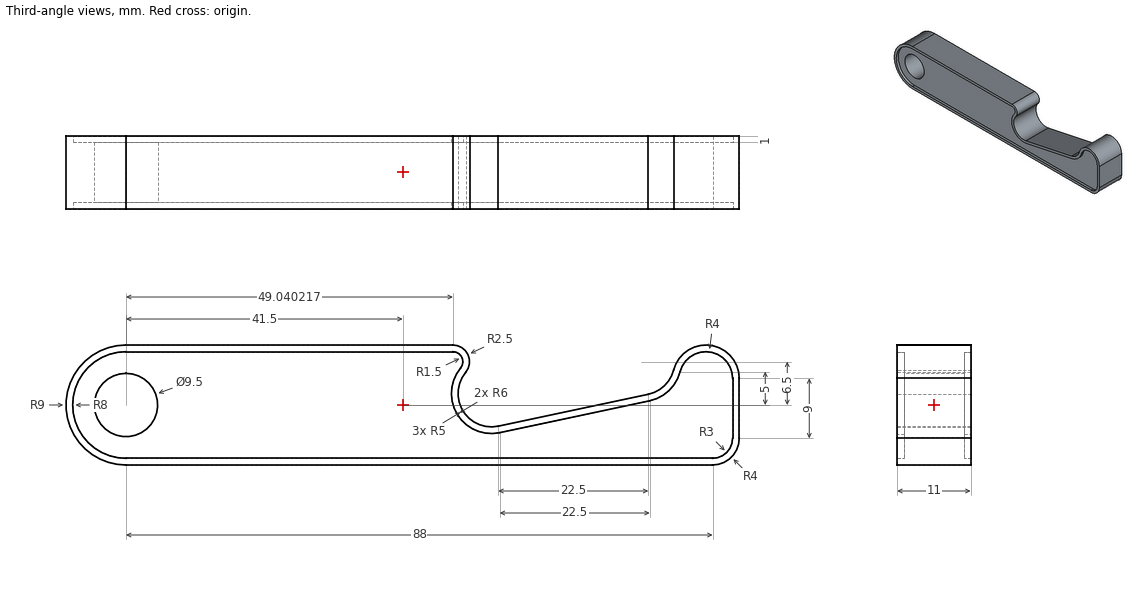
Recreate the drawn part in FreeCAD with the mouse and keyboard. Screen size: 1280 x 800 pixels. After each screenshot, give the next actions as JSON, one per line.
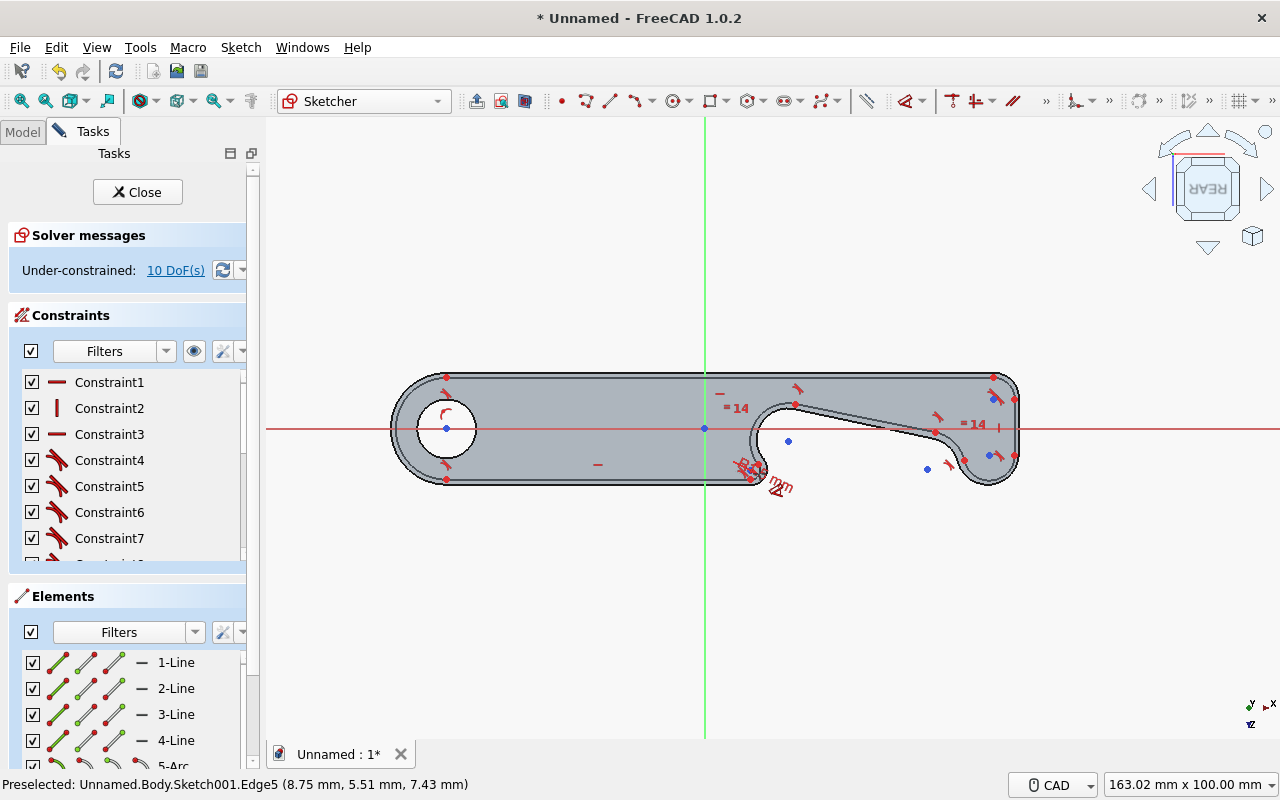
{"action": "left_click", "coordinate": [769, 409]}
{"action": "left_click", "coordinate": [728, 406]}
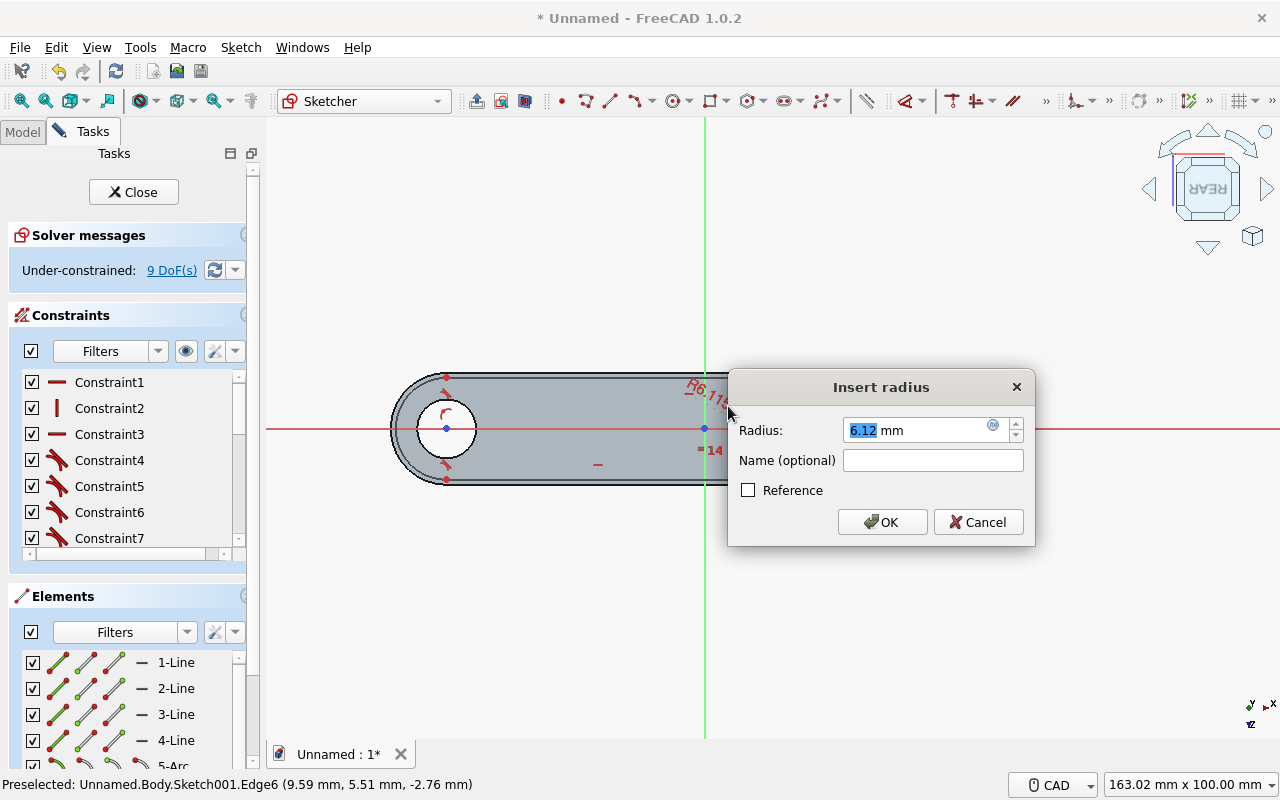
{"action": "type", "text": "6"}
{"action": "key", "text": "Return"}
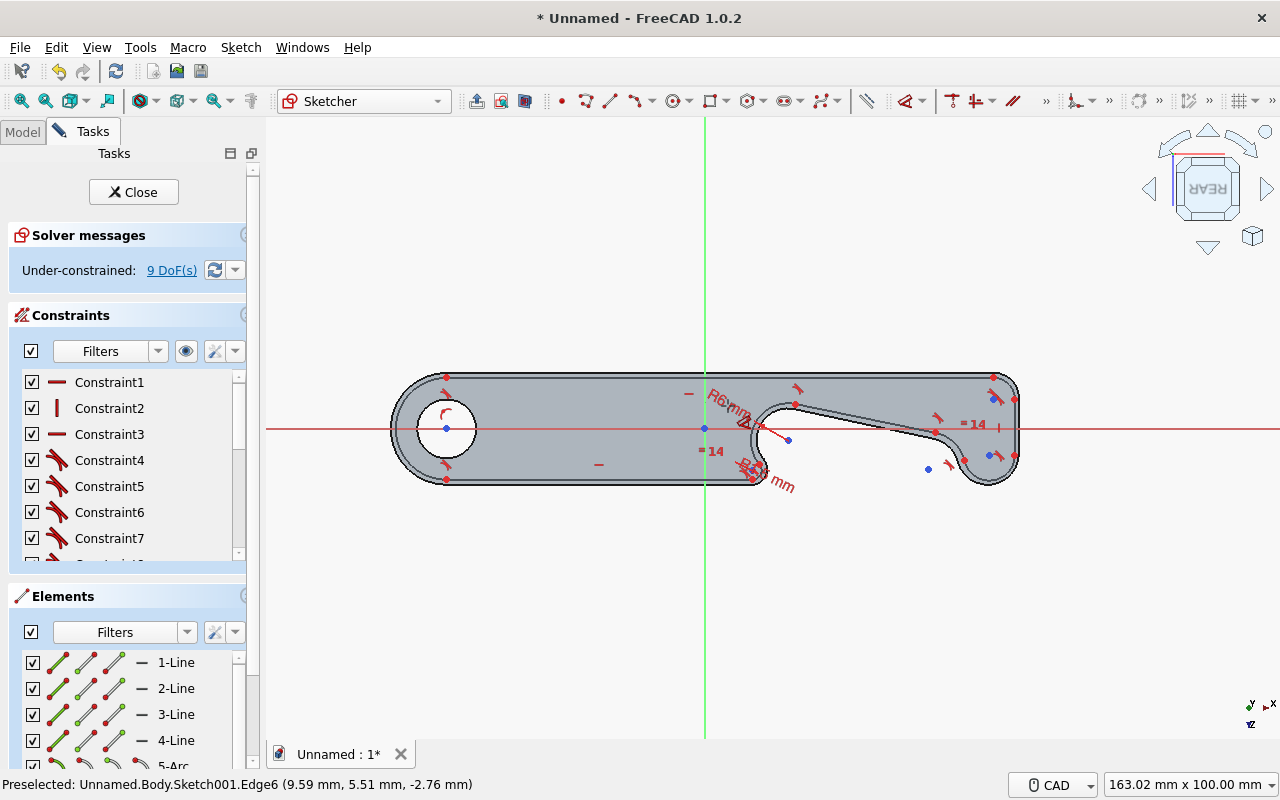
{"action": "scroll", "coordinate": [978, 478], "scroll_direction": "up", "scroll_amount": 3}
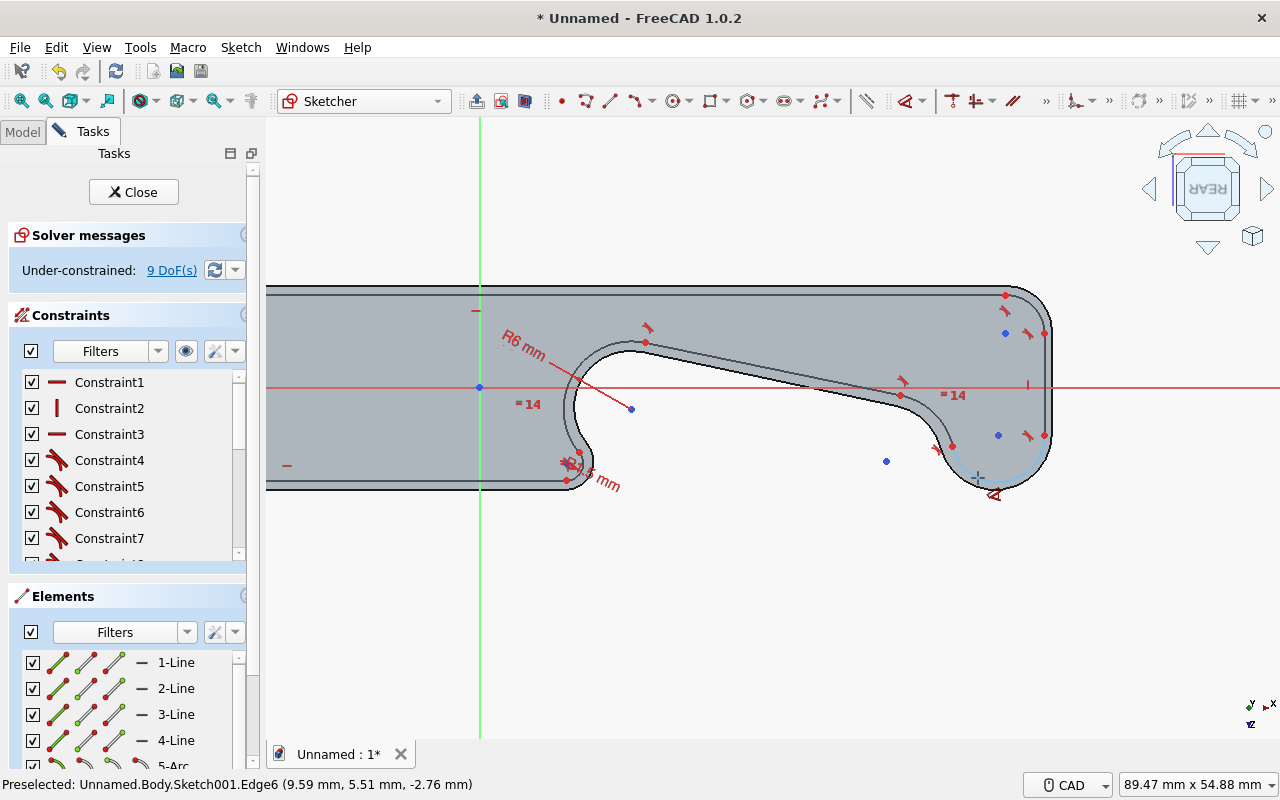
{"action": "left_click", "coordinate": [977, 477]}
{"action": "left_click", "coordinate": [962, 505]}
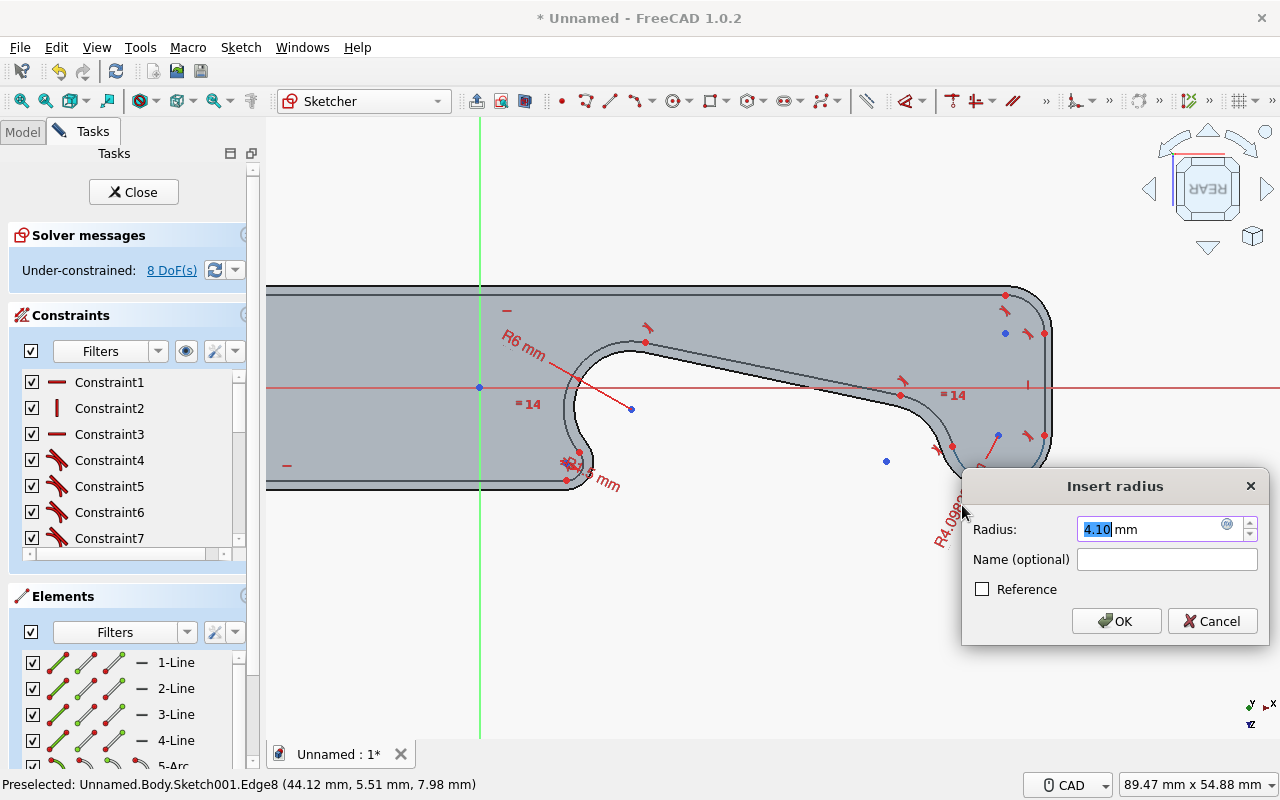
{"action": "type", "text": "4"}
{"action": "key", "text": "Return"}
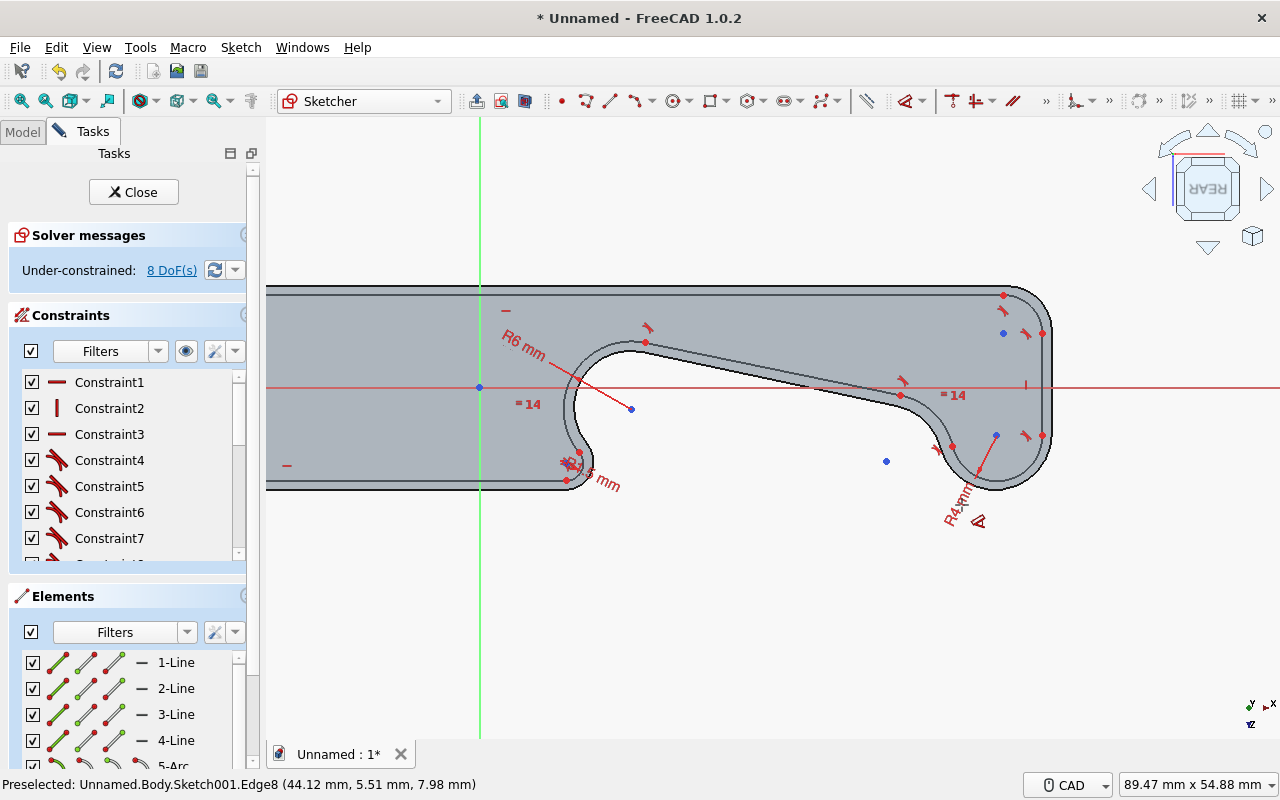
{"action": "left_click", "coordinate": [1038, 316]}
{"action": "left_click", "coordinate": [1066, 301]}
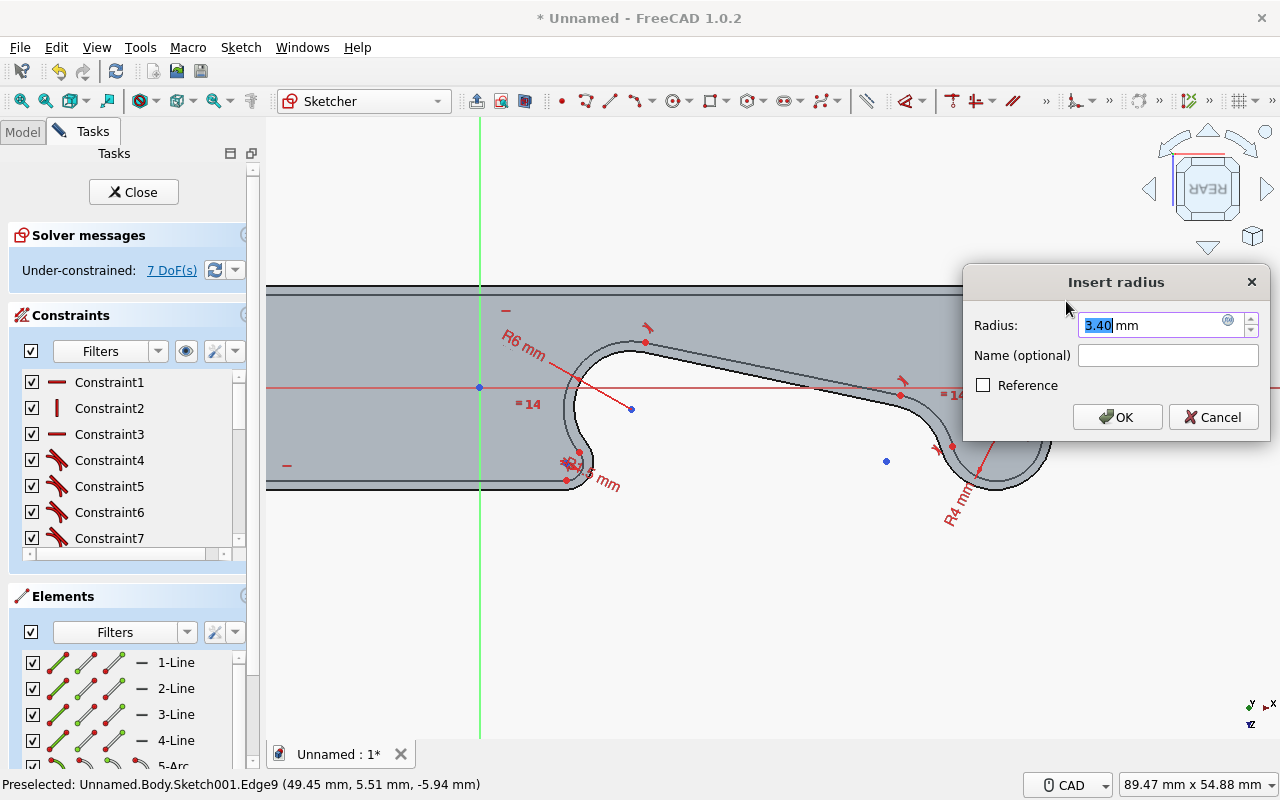
{"action": "type", "text": "3"}
{"action": "key", "text": "Return"}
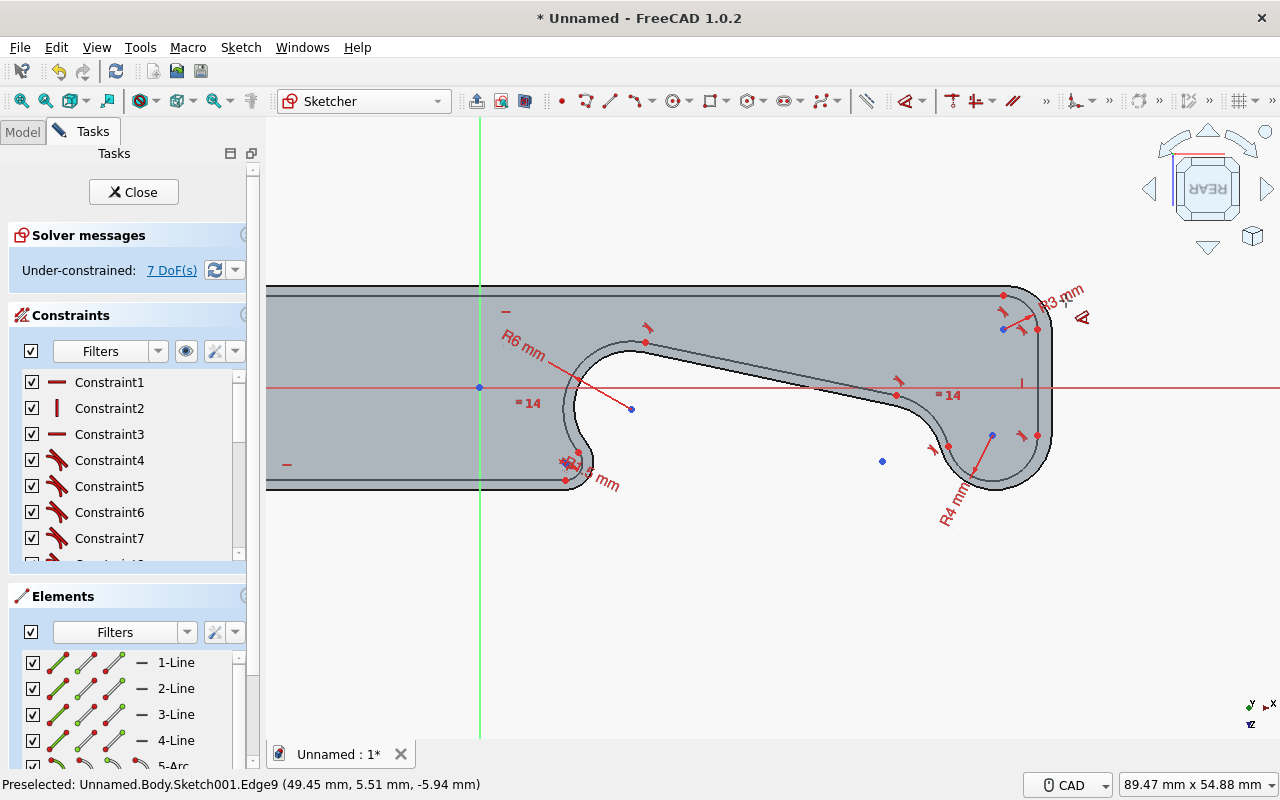
{"action": "scroll", "coordinate": [978, 477], "scroll_direction": "down", "scroll_amount": 3}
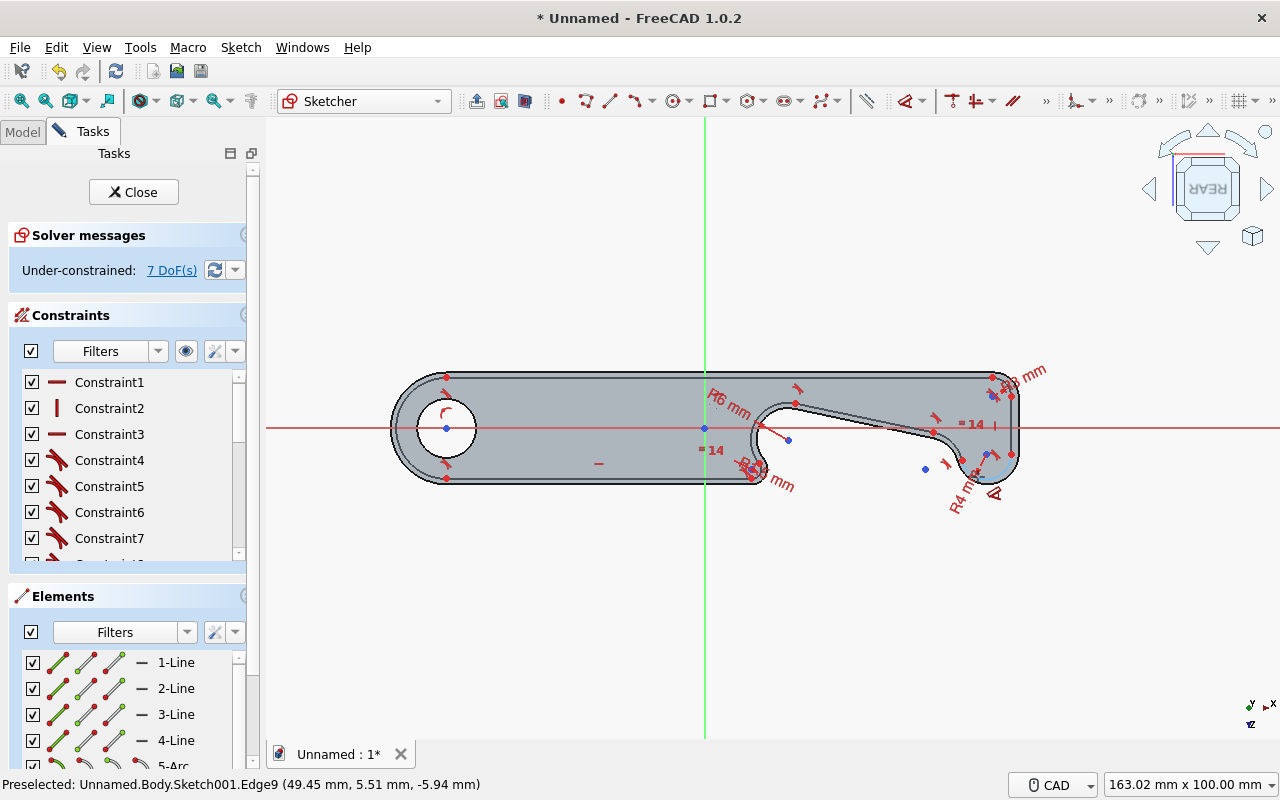
{"action": "left_click", "coordinate": [406, 399]}
{"action": "left_click", "coordinate": [380, 380]}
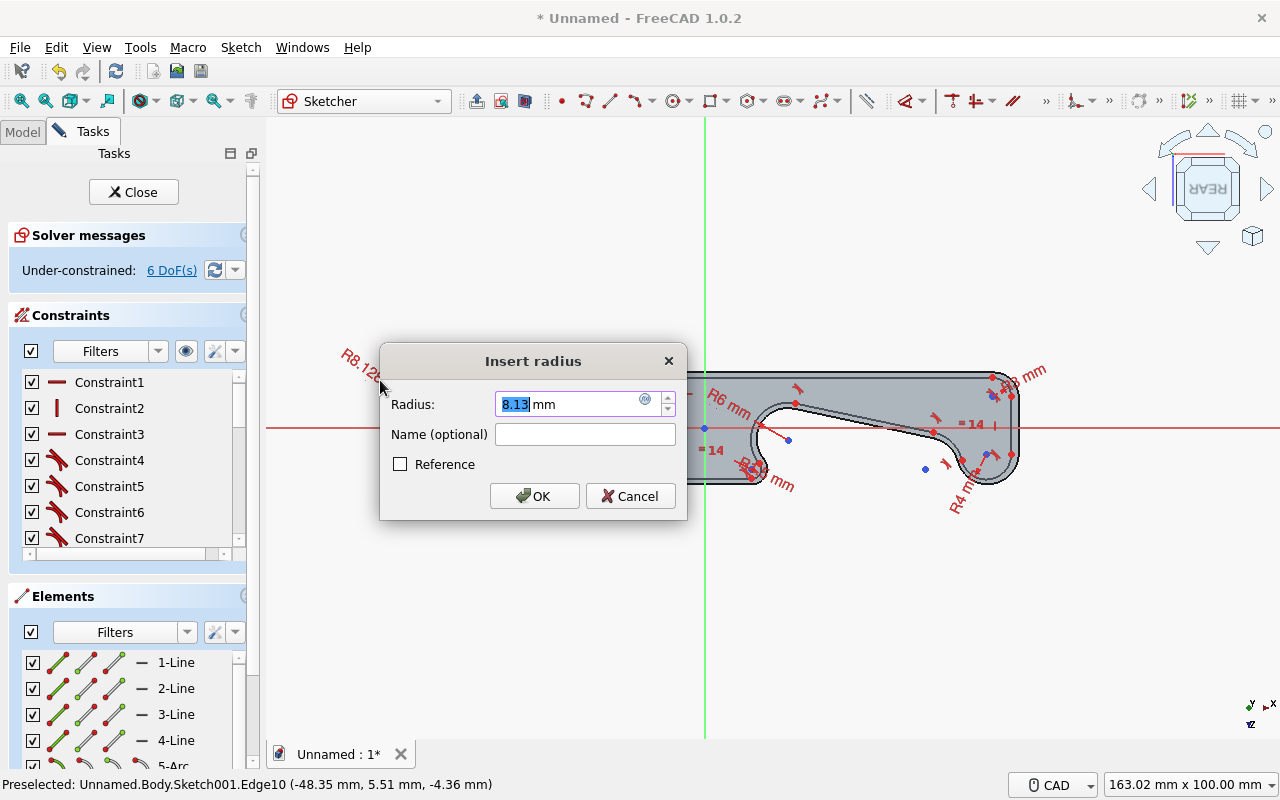
{"action": "type", "text": "8"}
{"action": "key", "text": "Return"}